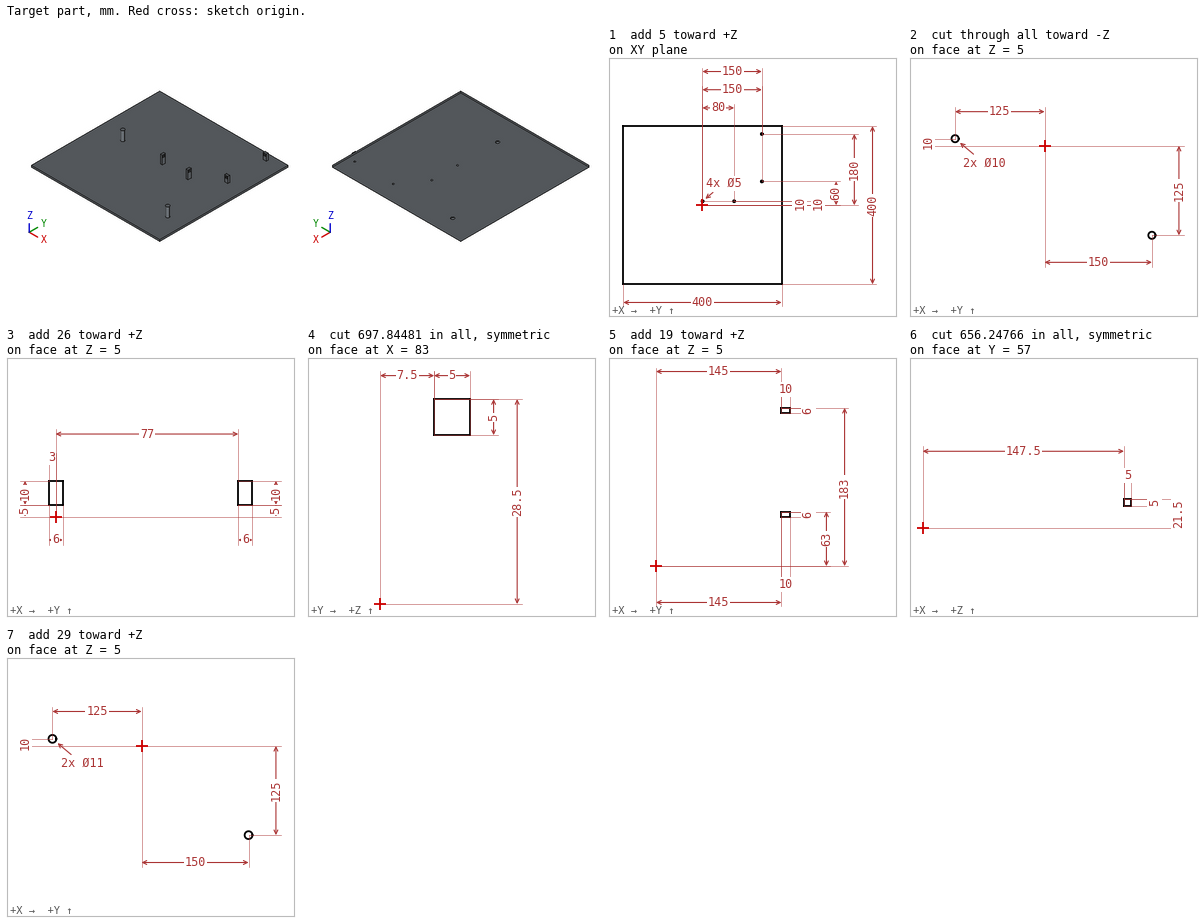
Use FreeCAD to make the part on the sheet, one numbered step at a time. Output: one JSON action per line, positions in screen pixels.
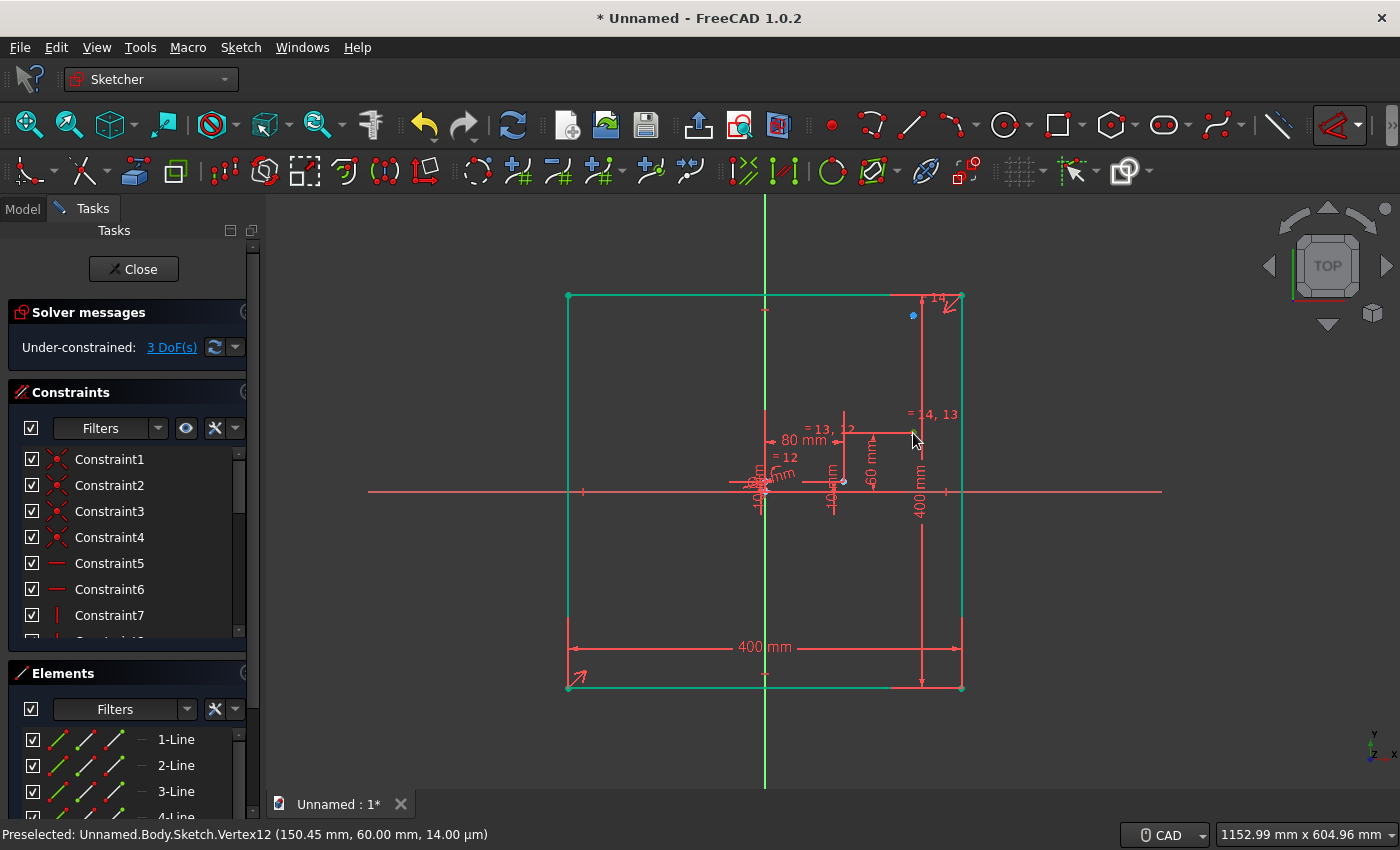
{"action": "key", "text": "l"}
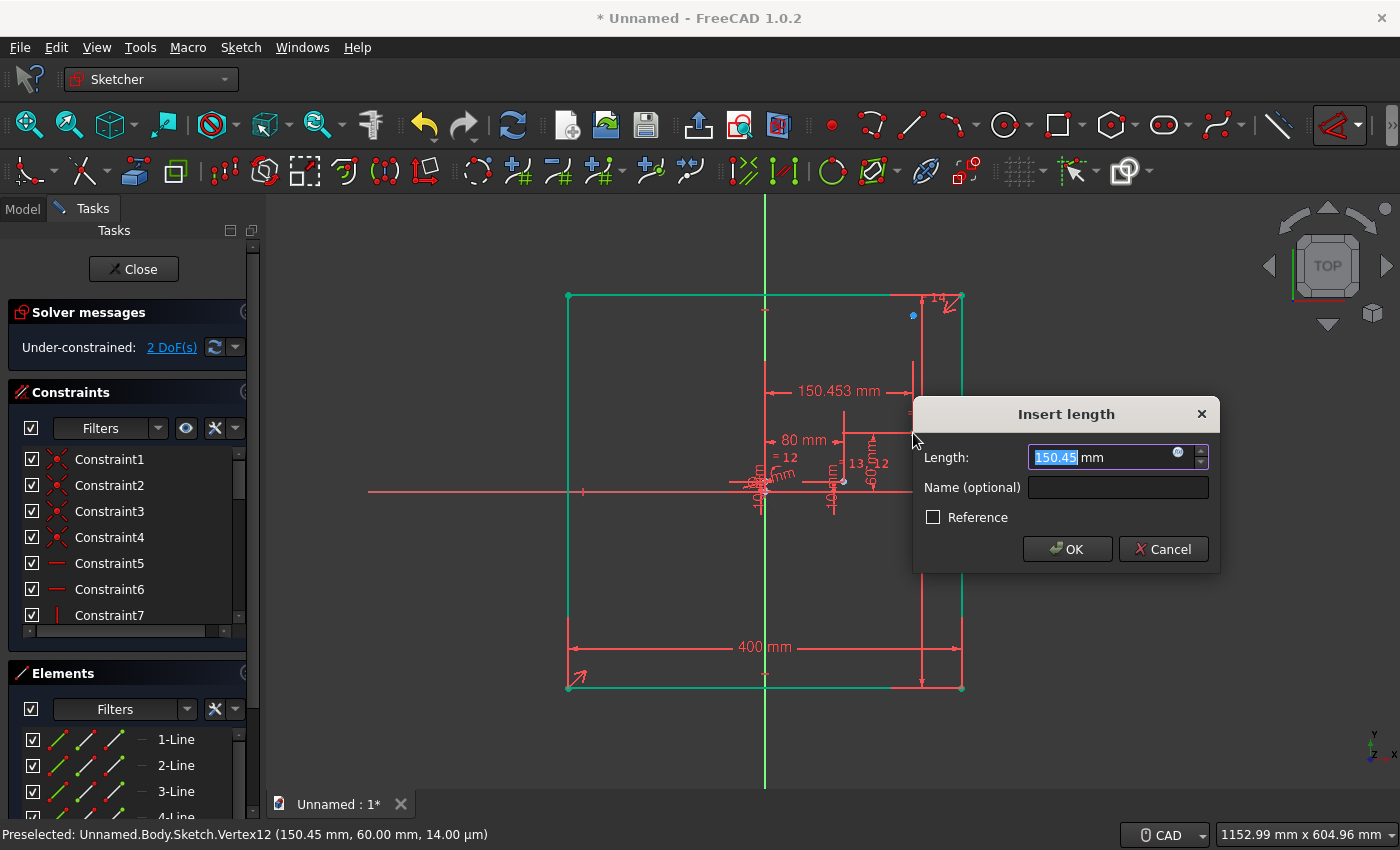
{"action": "type", "text": "150"}
{"action": "key", "text": "Return"}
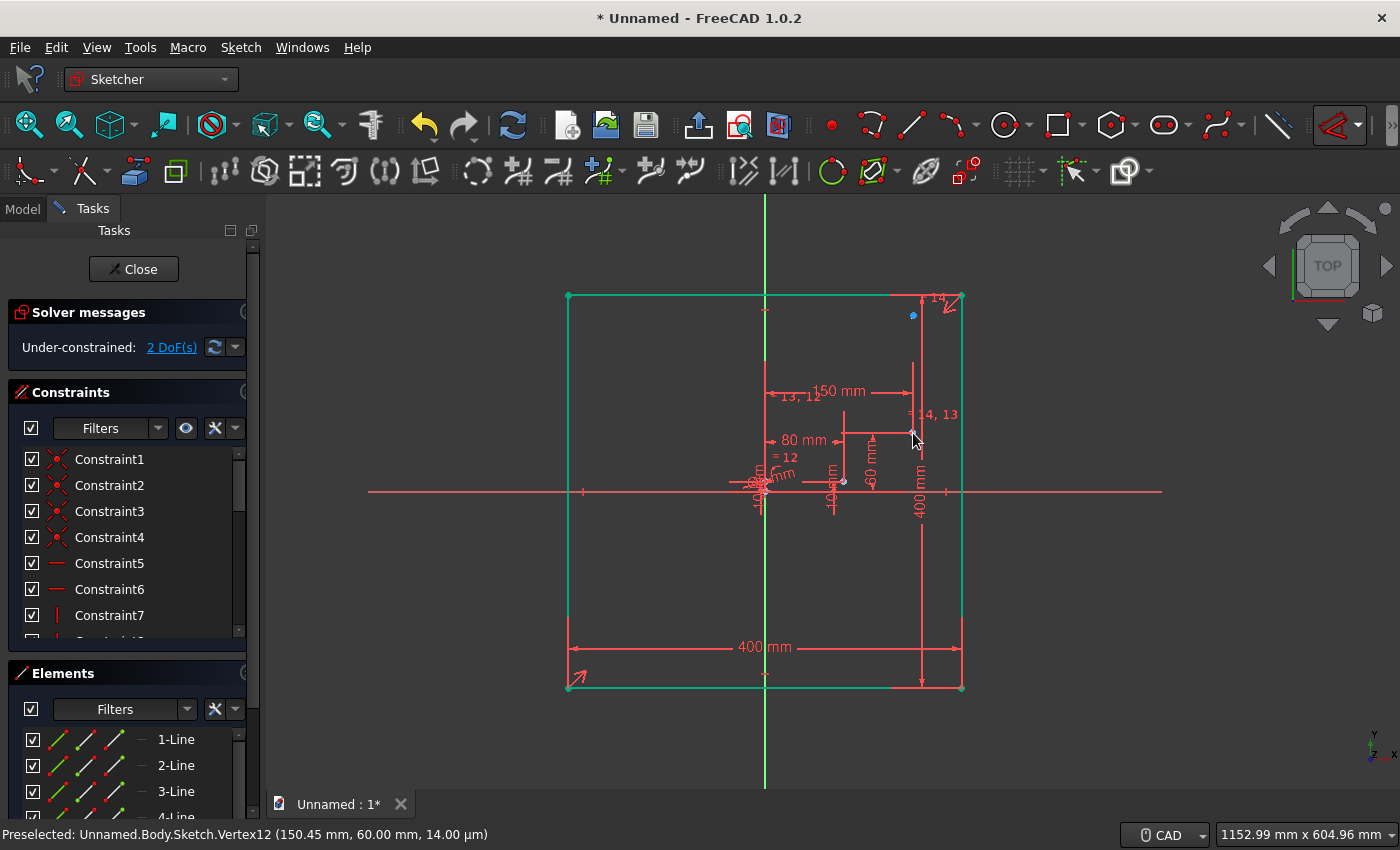
{"action": "left_click", "coordinate": [913, 316]}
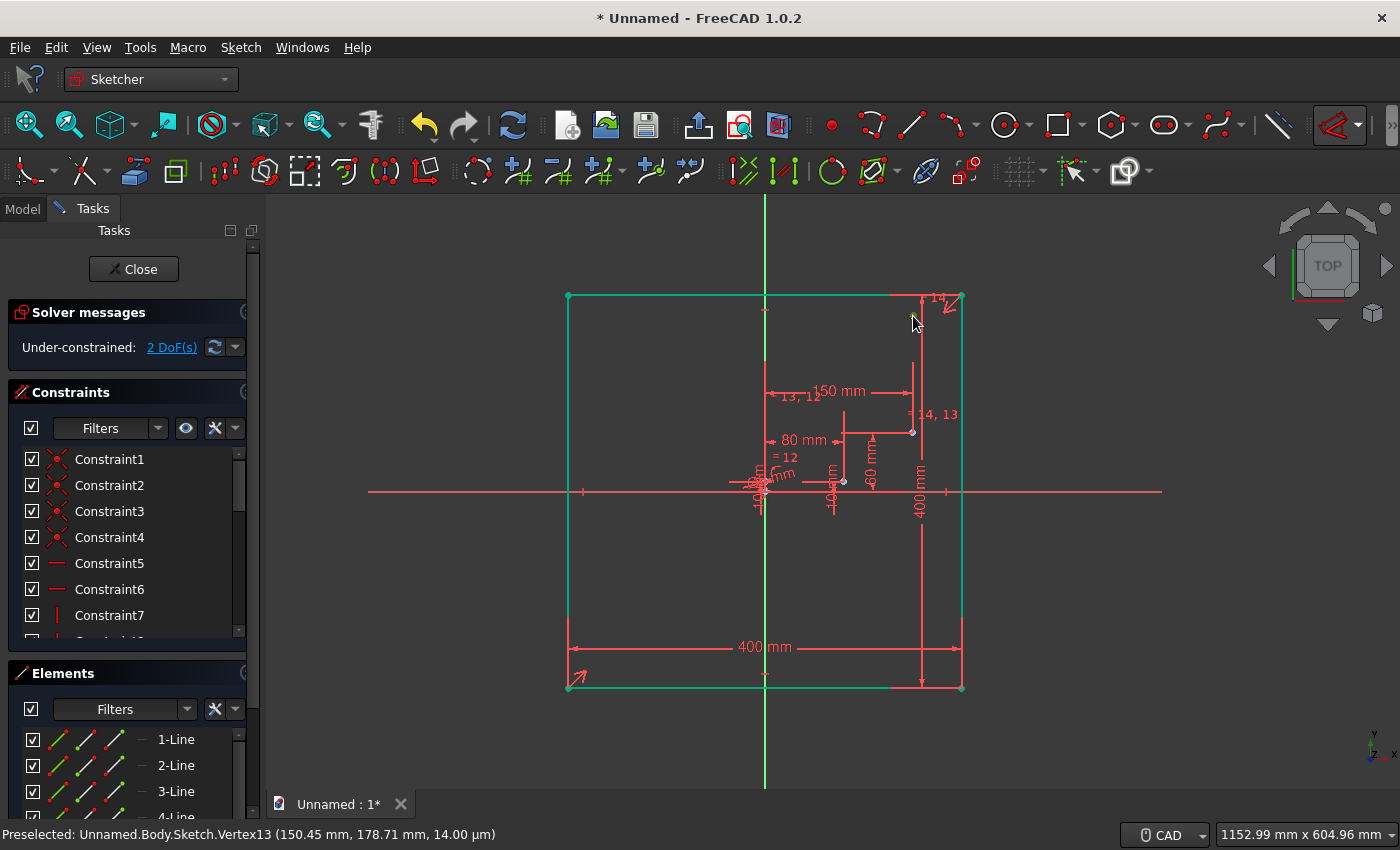
{"action": "key", "text": "l"}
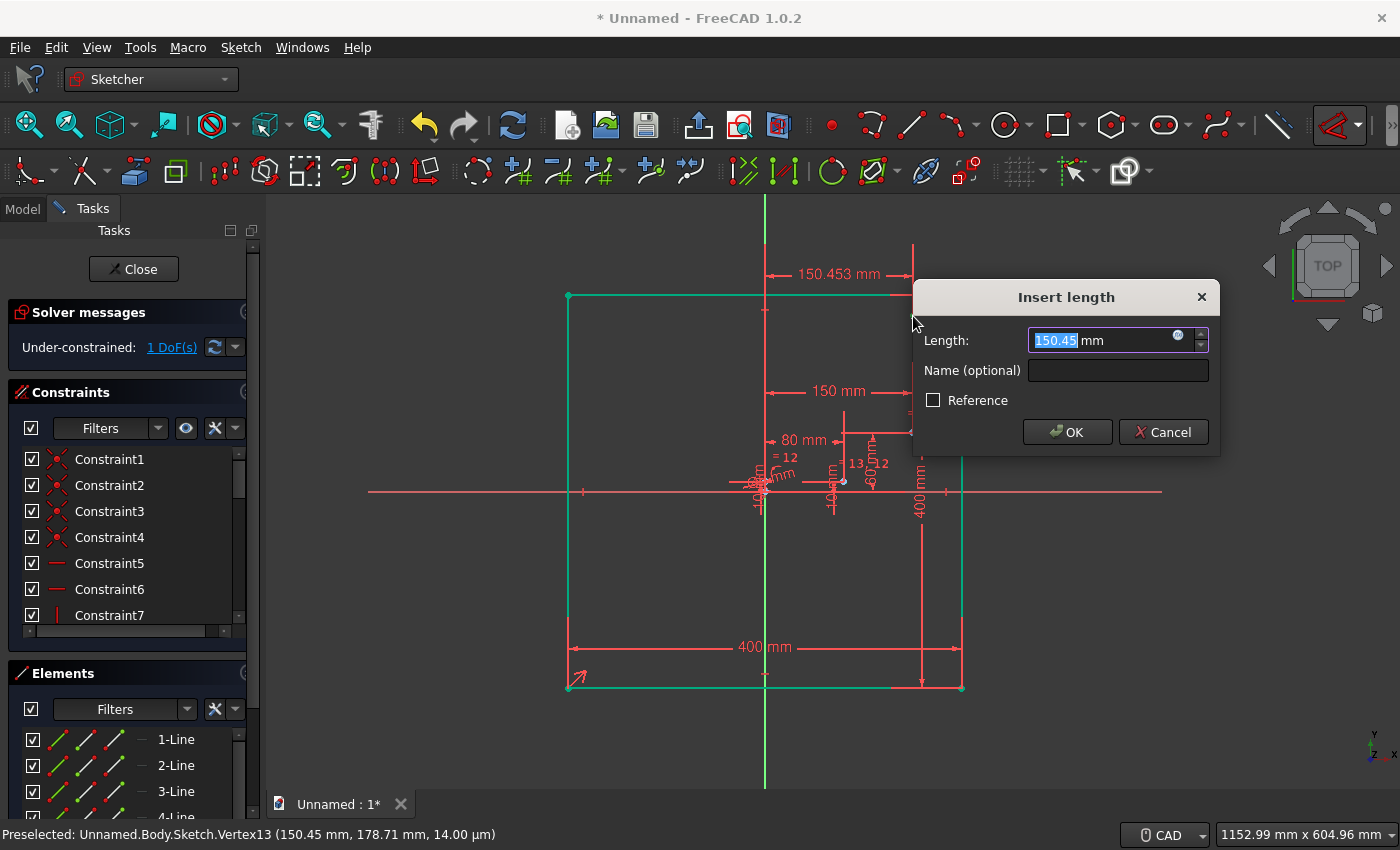
{"action": "type", "text": "150"}
{"action": "key", "text": "Return"}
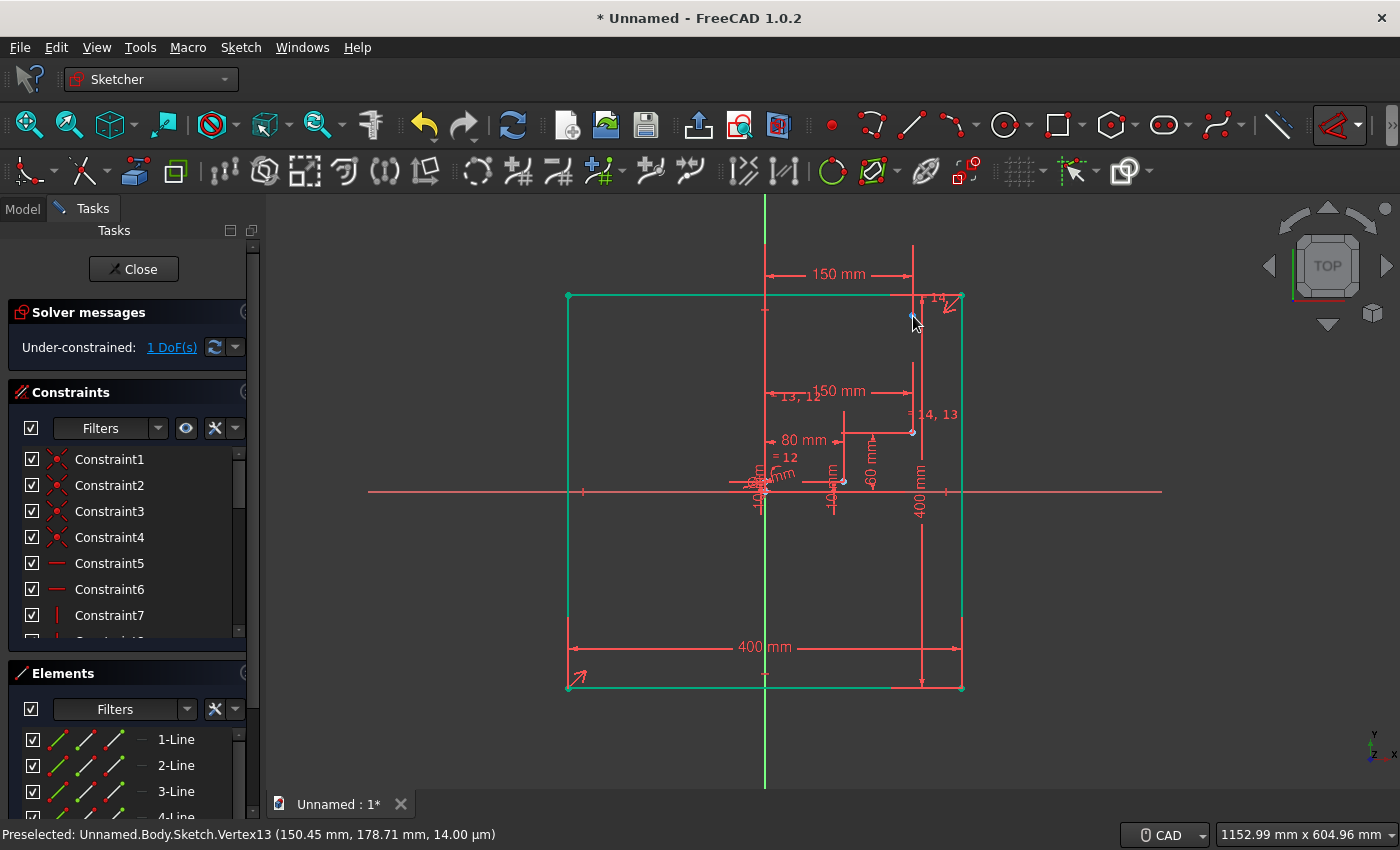
{"action": "left_click", "coordinate": [913, 316]}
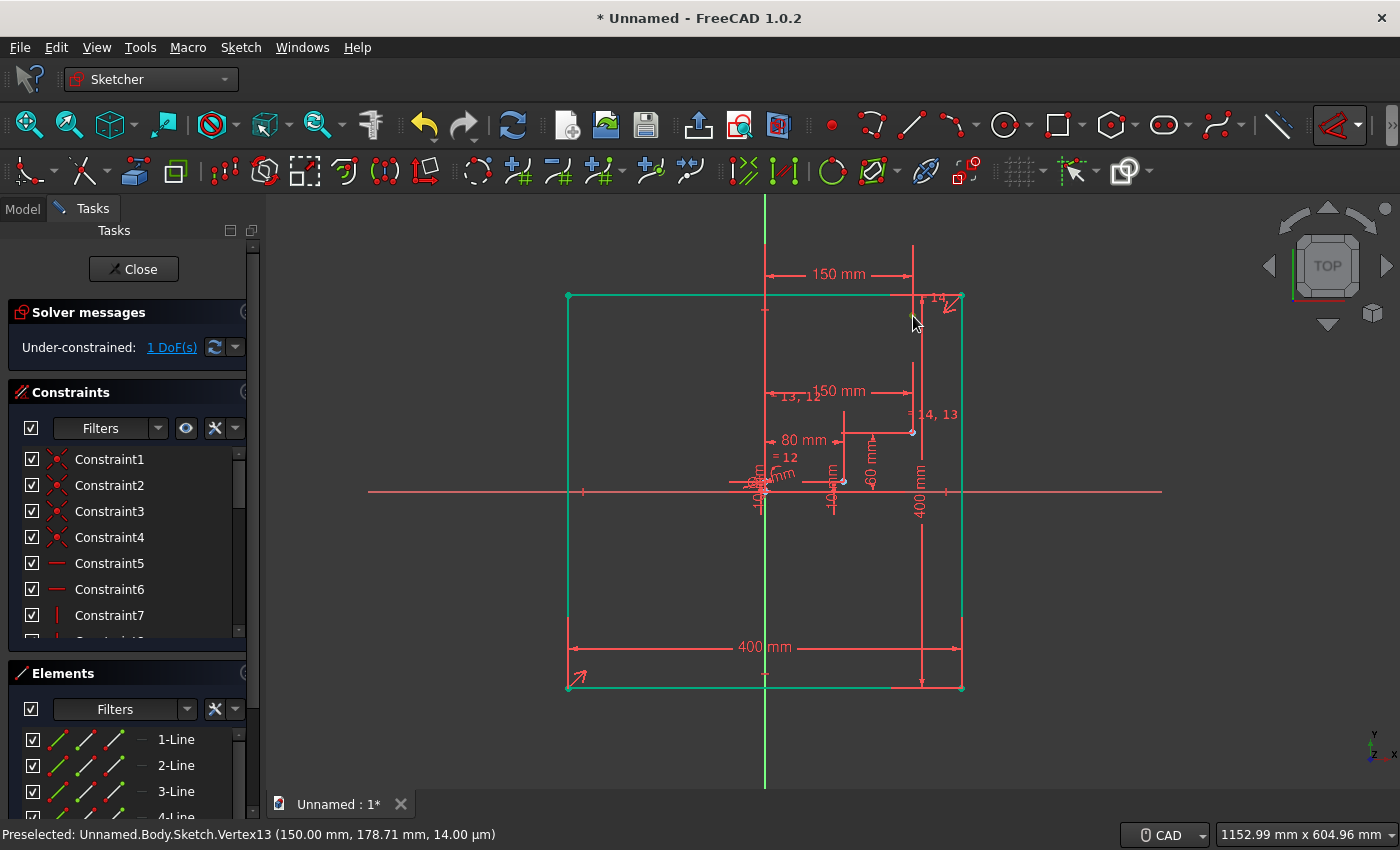
{"action": "key", "text": "i"}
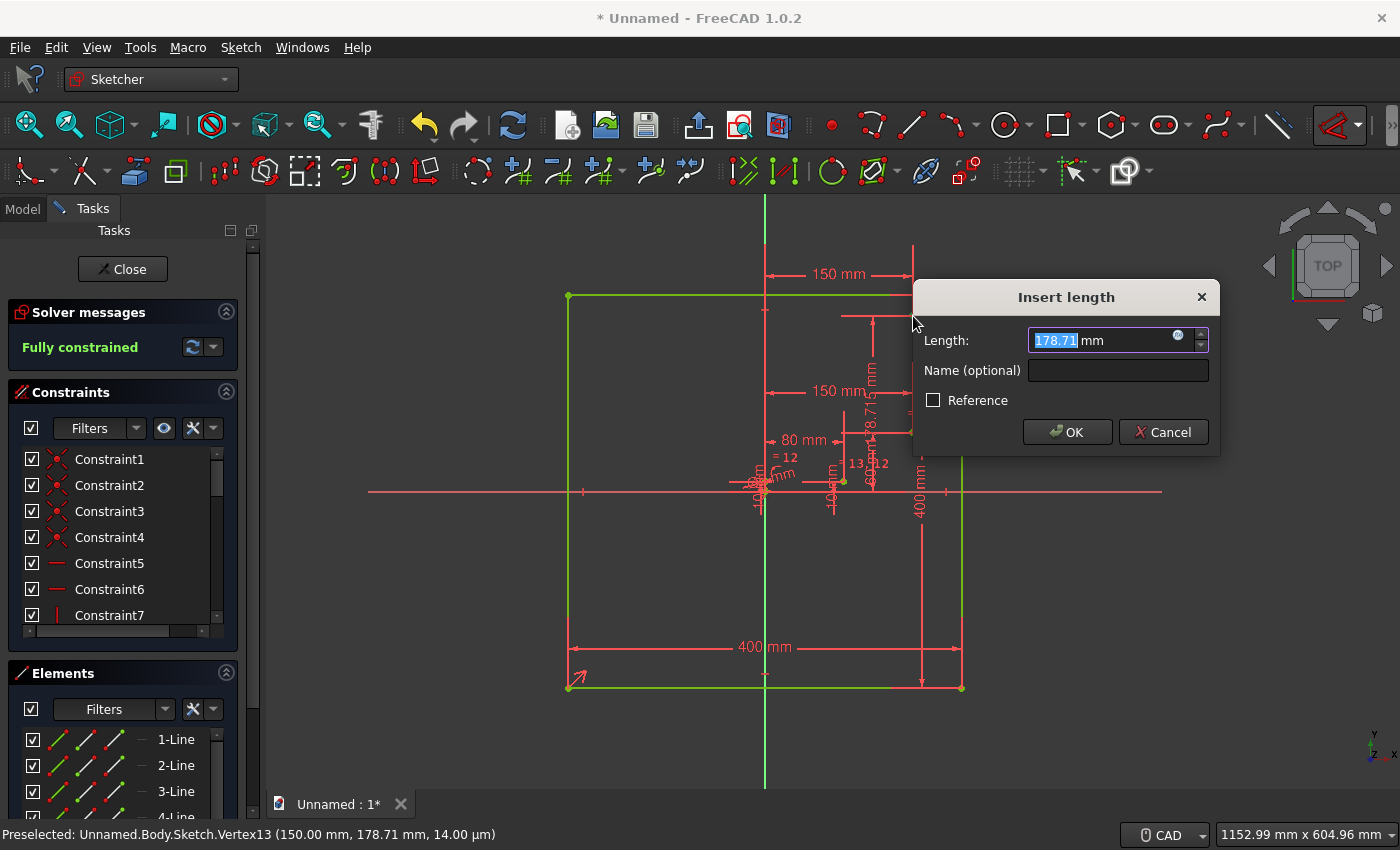
{"action": "type", "text": "180"}
{"action": "key", "text": "Return"}